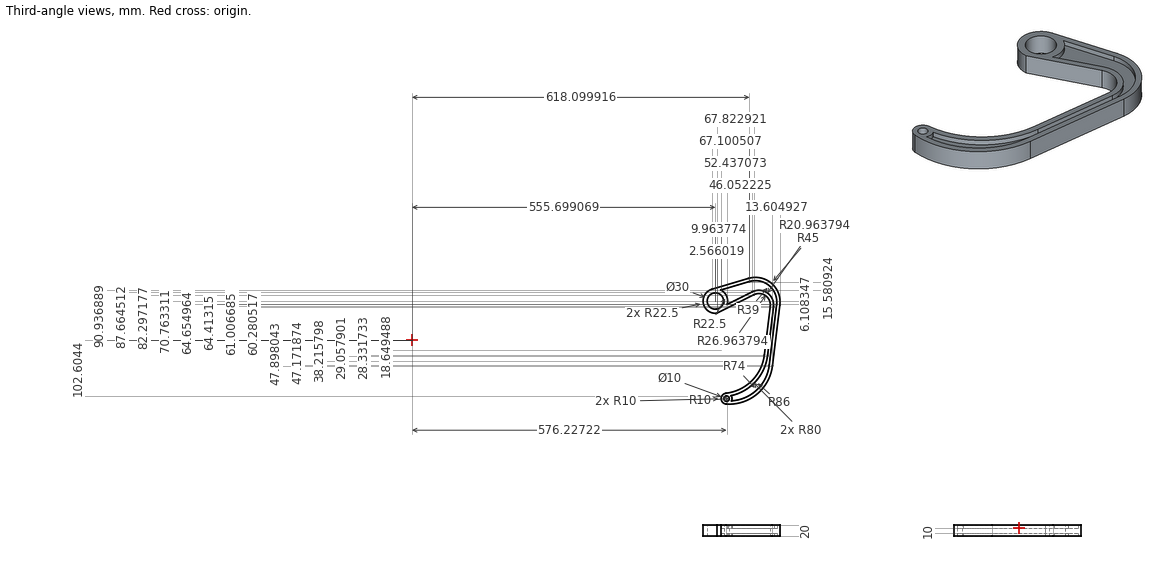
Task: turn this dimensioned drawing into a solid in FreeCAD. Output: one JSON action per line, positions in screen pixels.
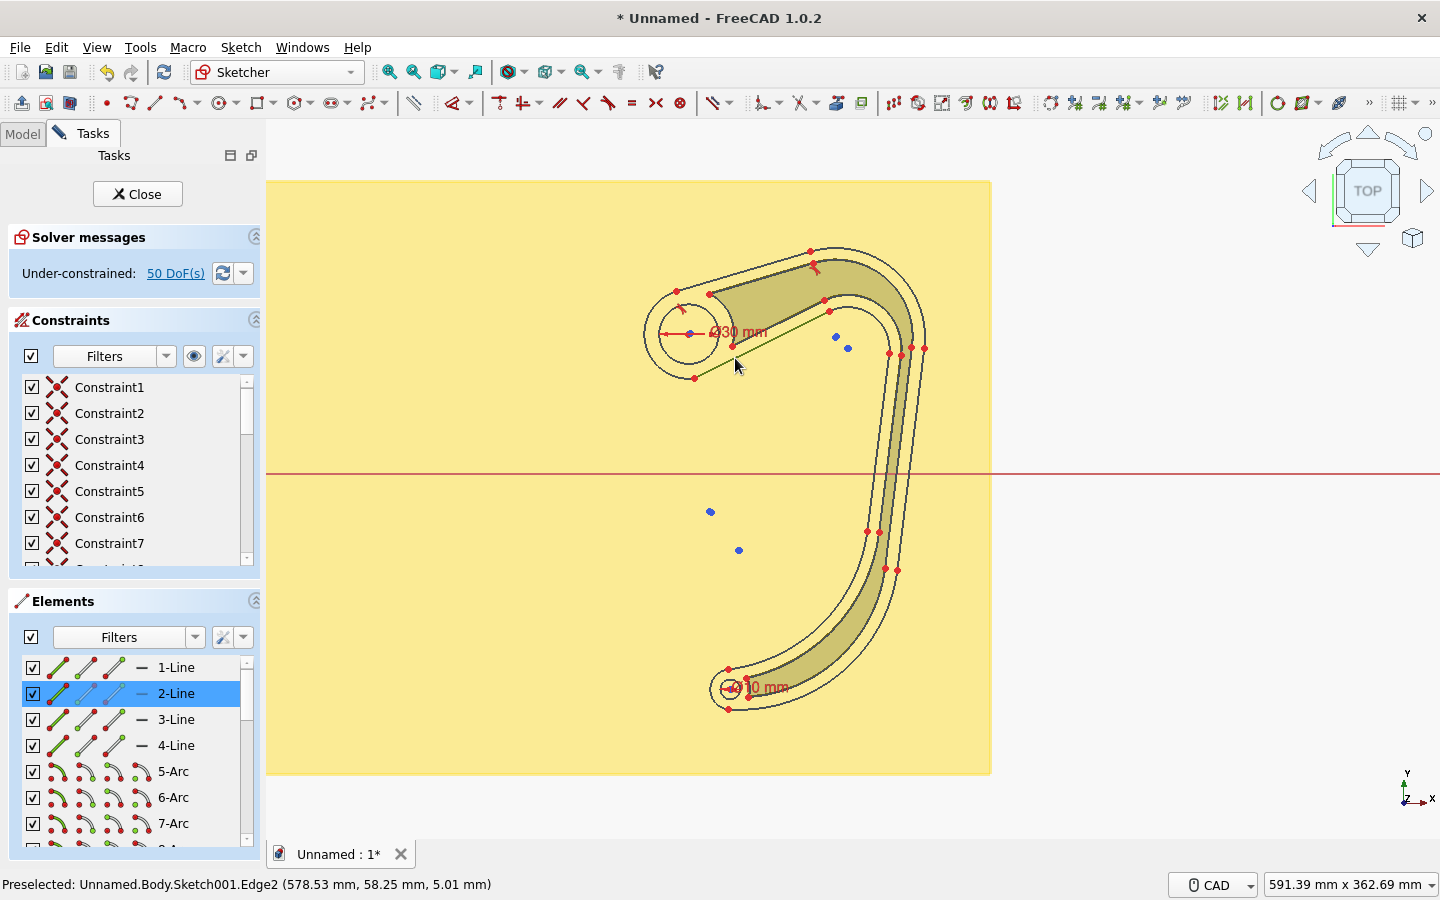
{"action": "left_click", "coordinate": [884, 328]}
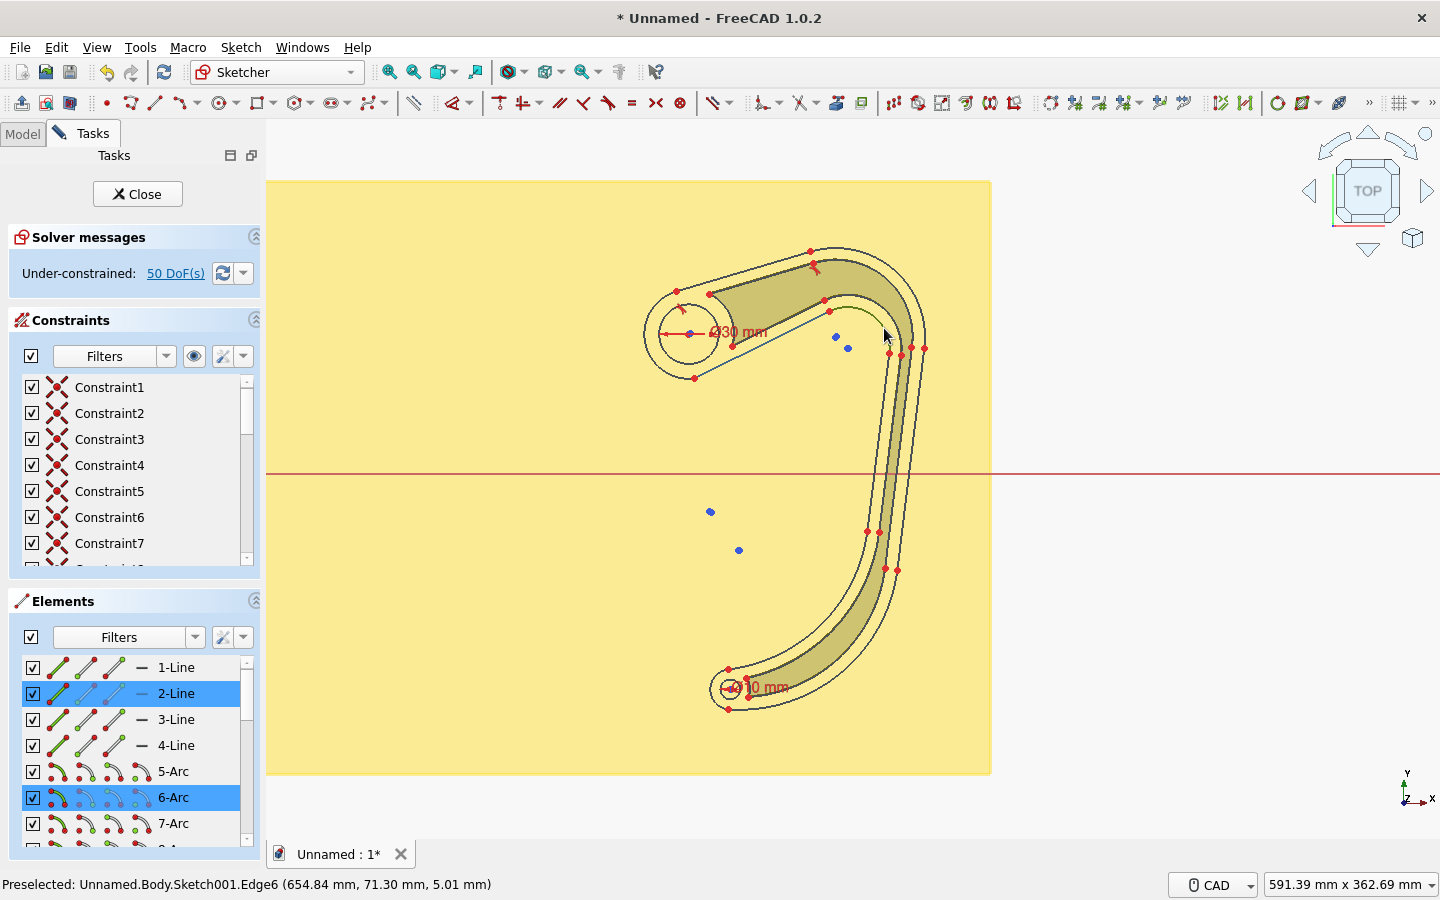
{"action": "left_click", "coordinate": [608, 104]}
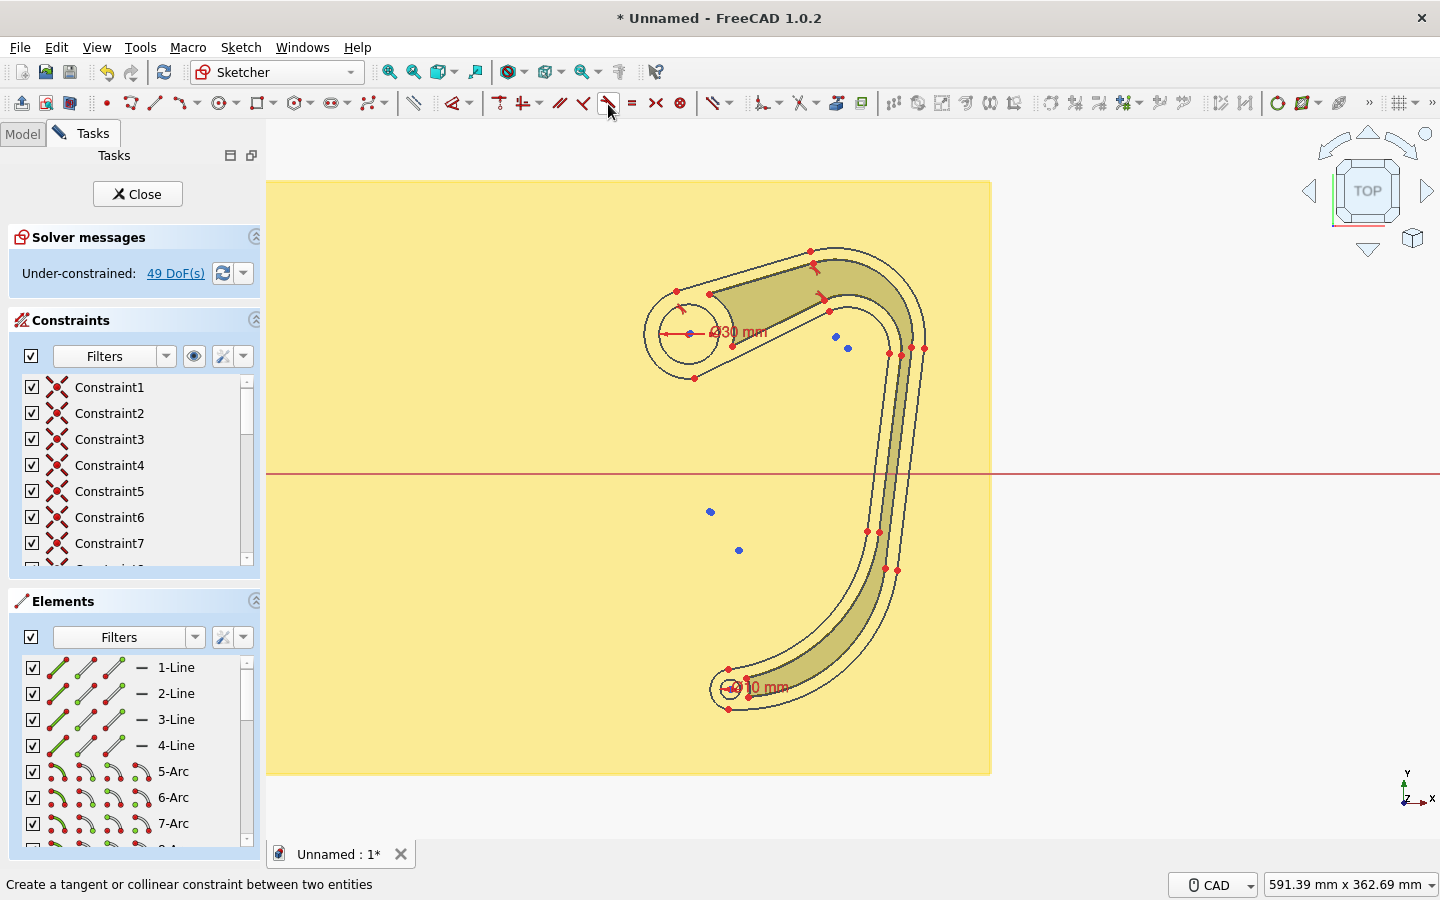
{"action": "left_click", "coordinate": [883, 407]}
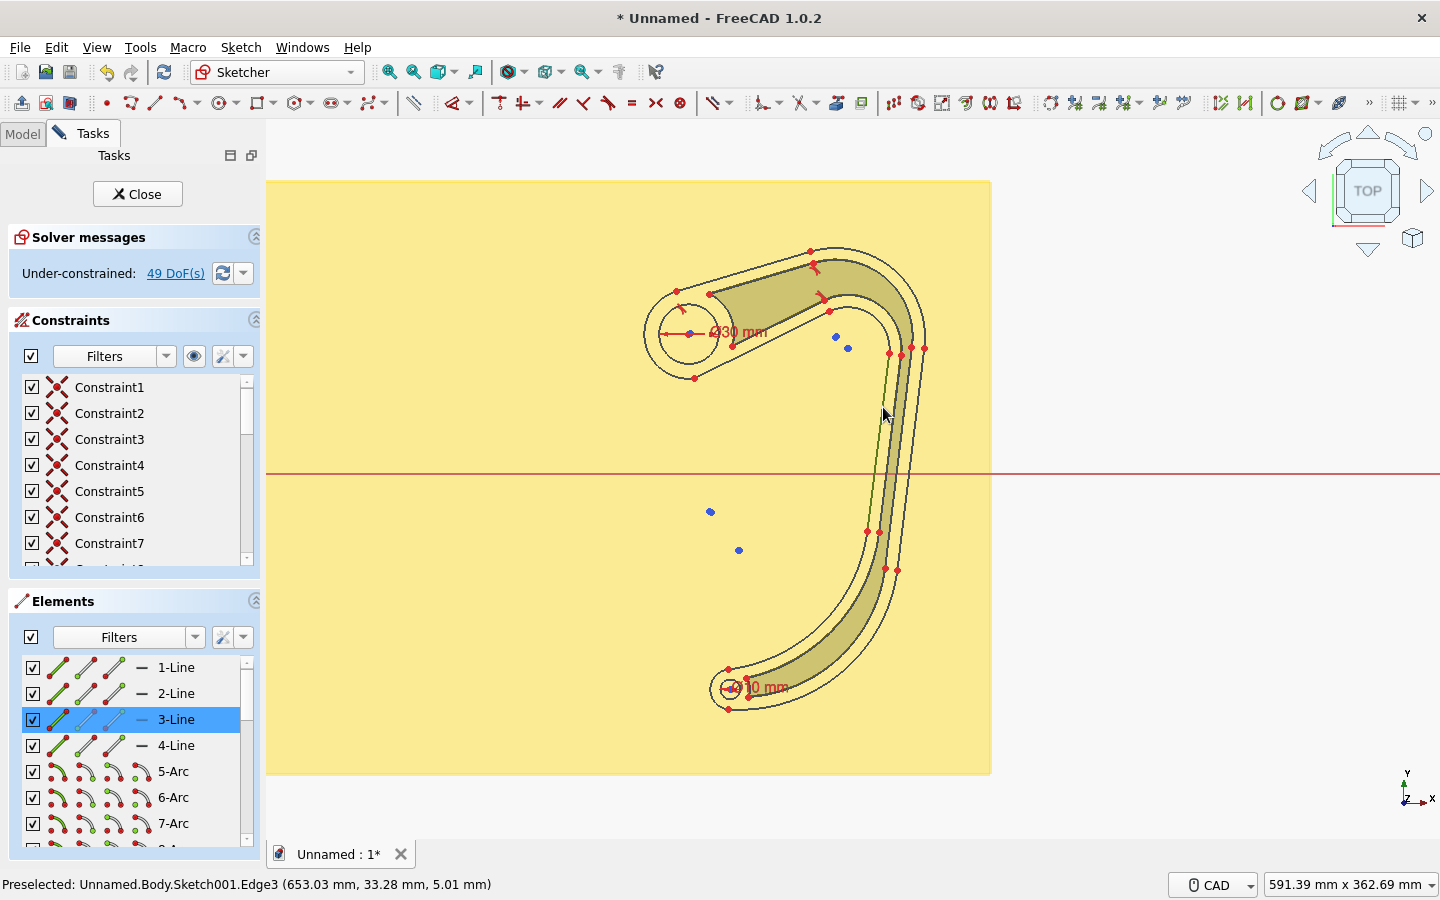
{"action": "left_click", "coordinate": [884, 328]}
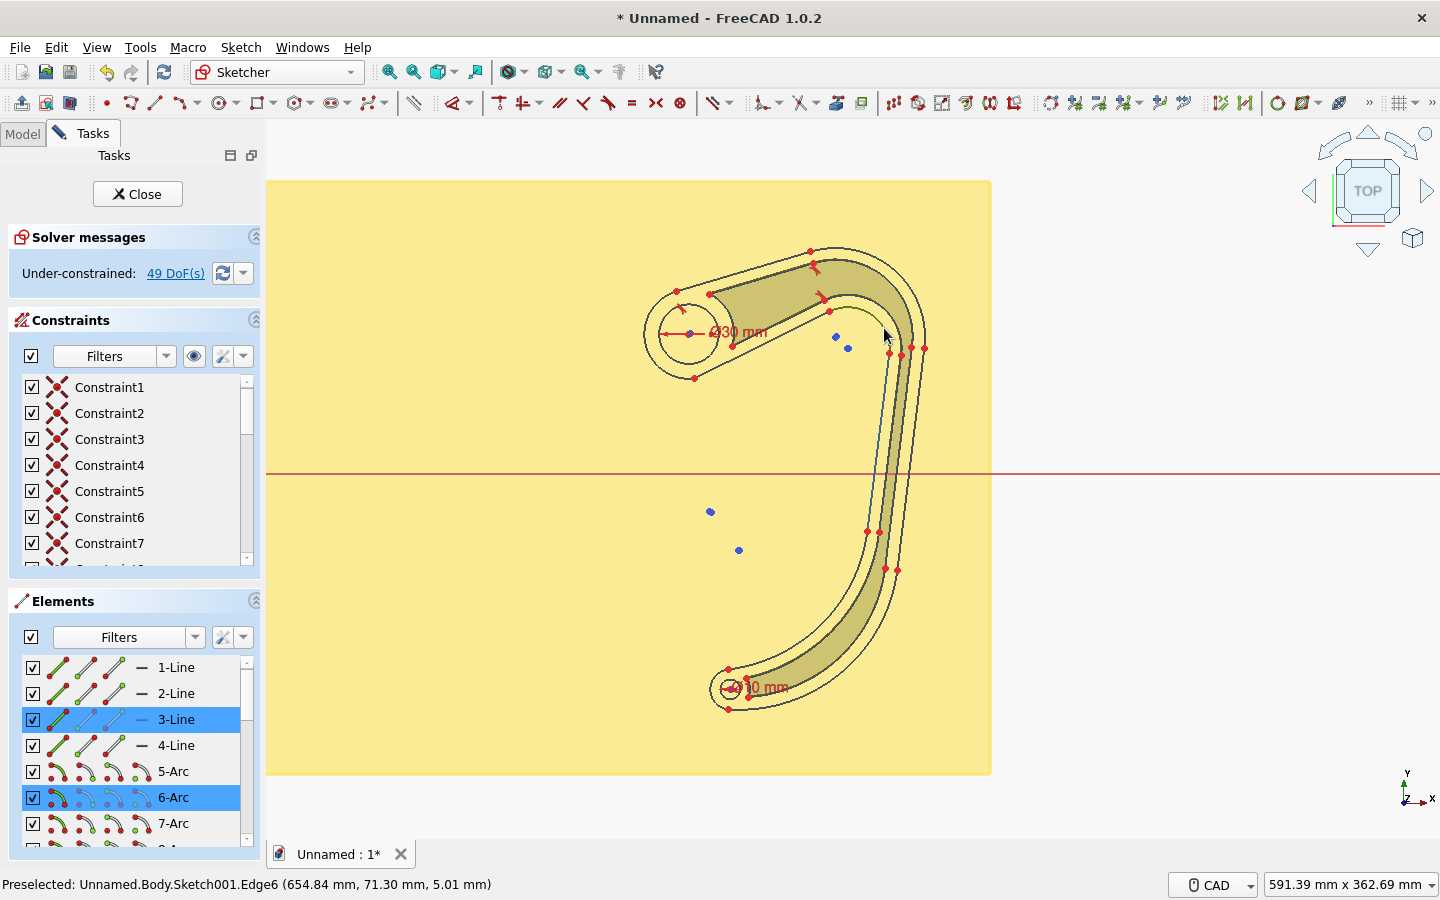
{"action": "left_click", "coordinate": [608, 104]}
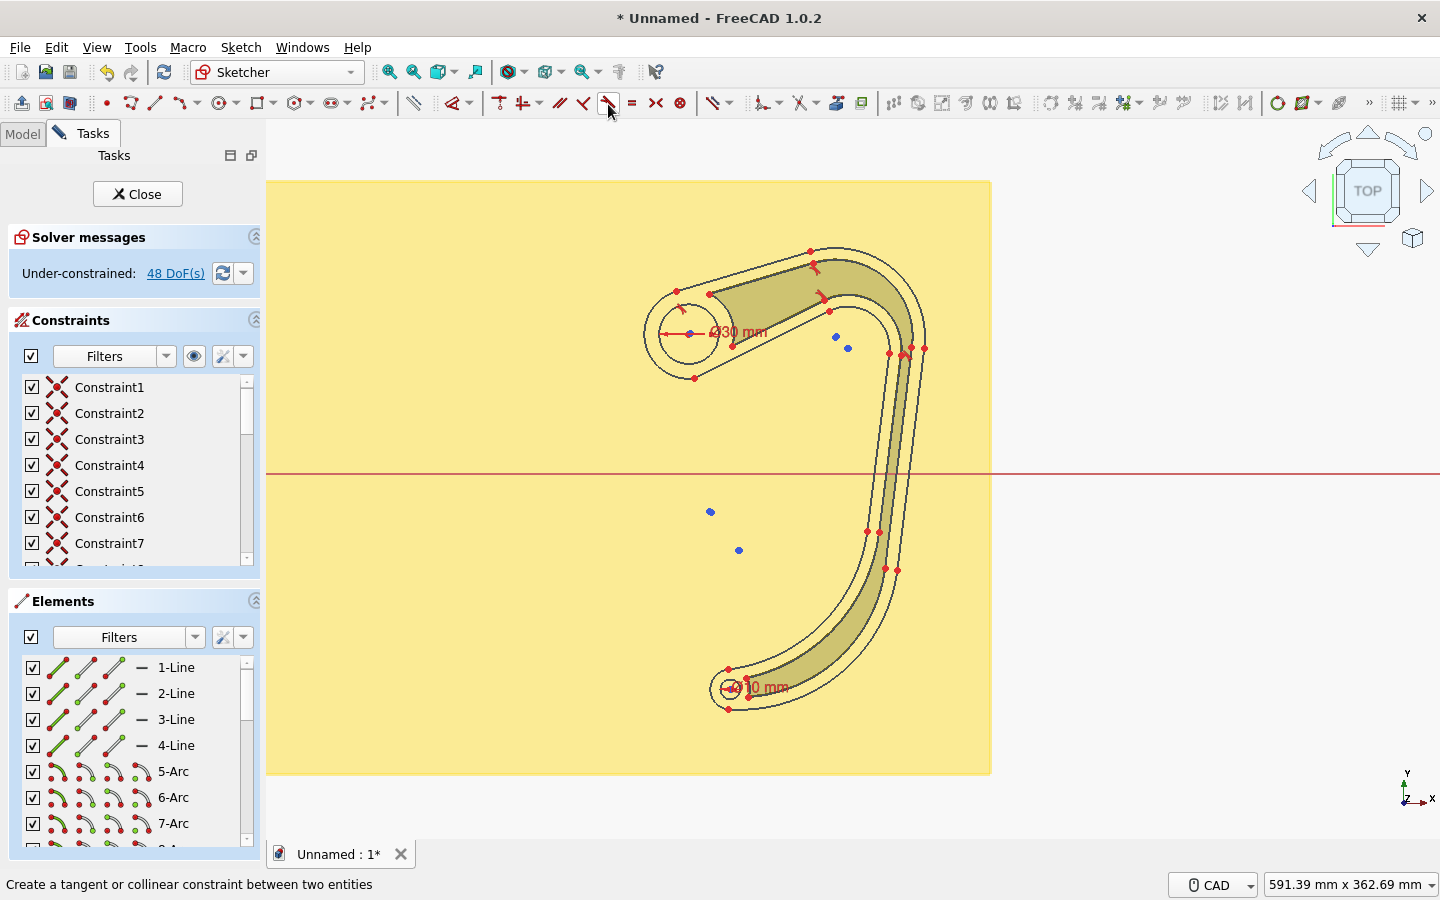
{"action": "left_click", "coordinate": [905, 504]}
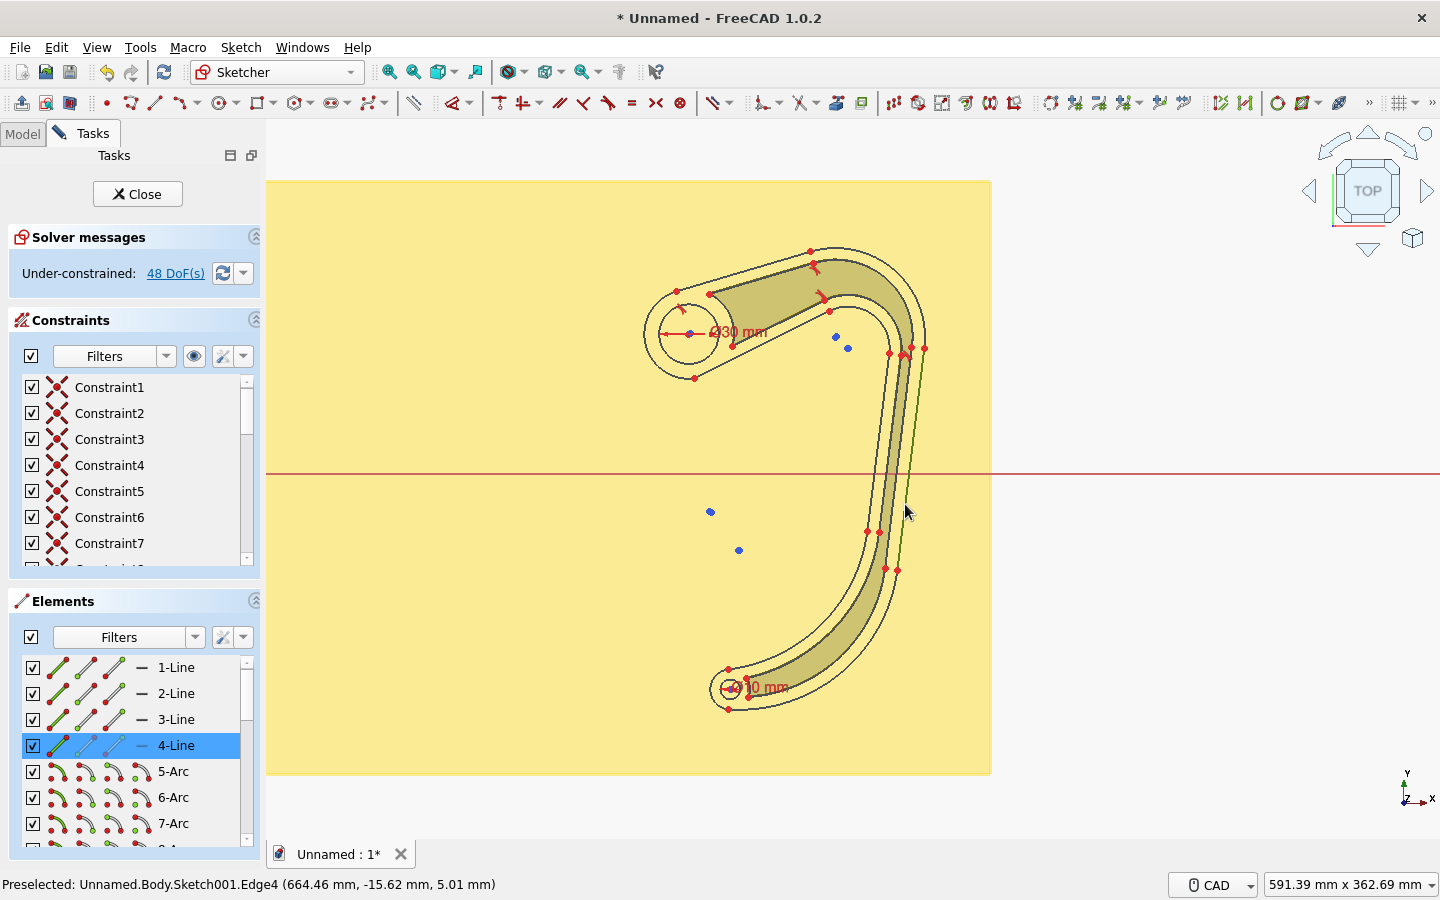
{"action": "left_click", "coordinate": [915, 297]}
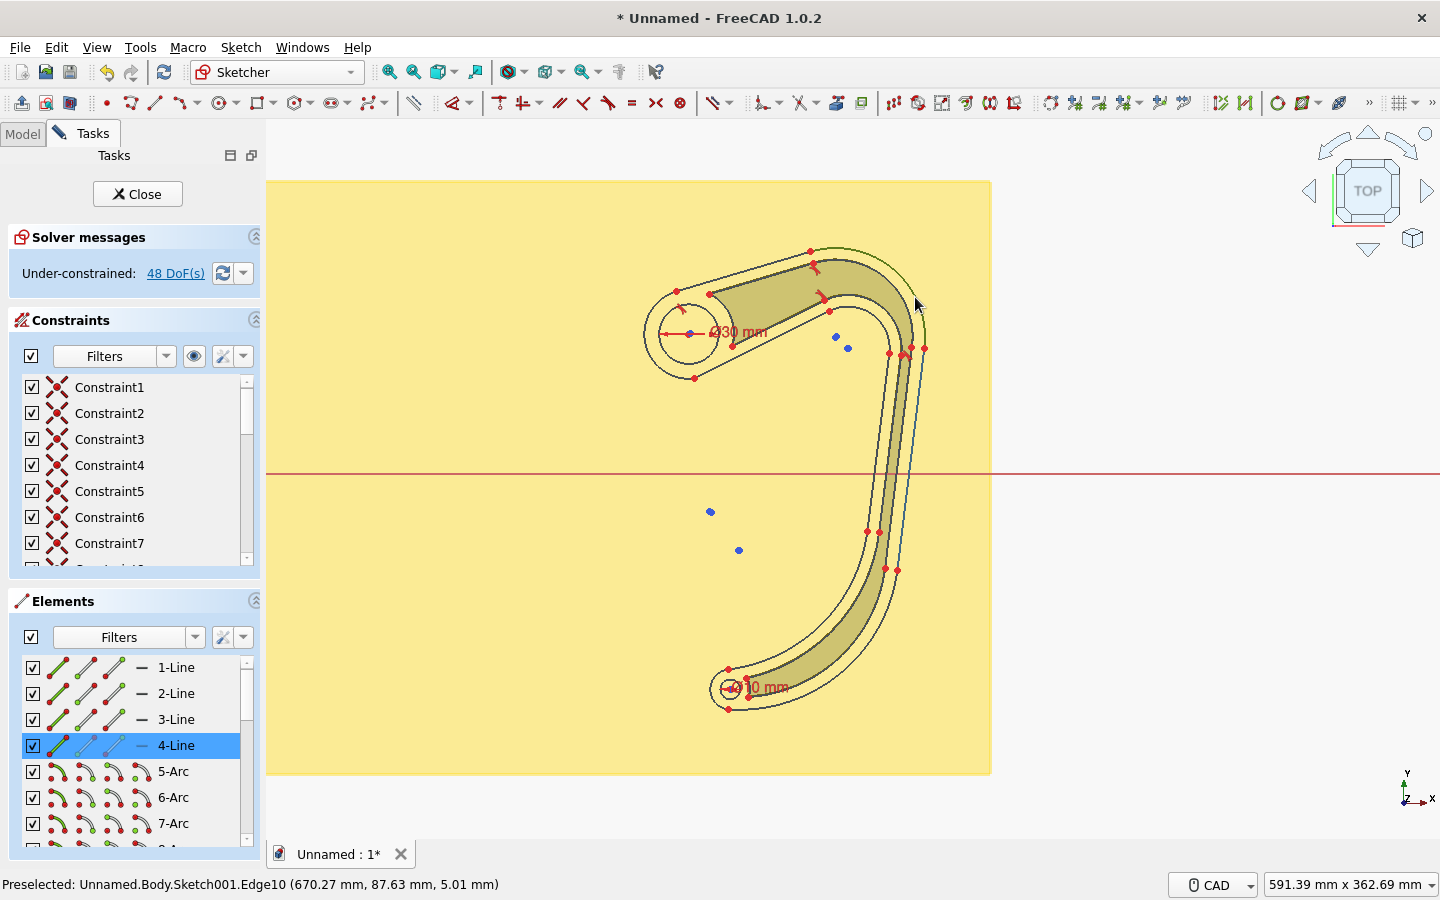
{"action": "key", "text": "t"}